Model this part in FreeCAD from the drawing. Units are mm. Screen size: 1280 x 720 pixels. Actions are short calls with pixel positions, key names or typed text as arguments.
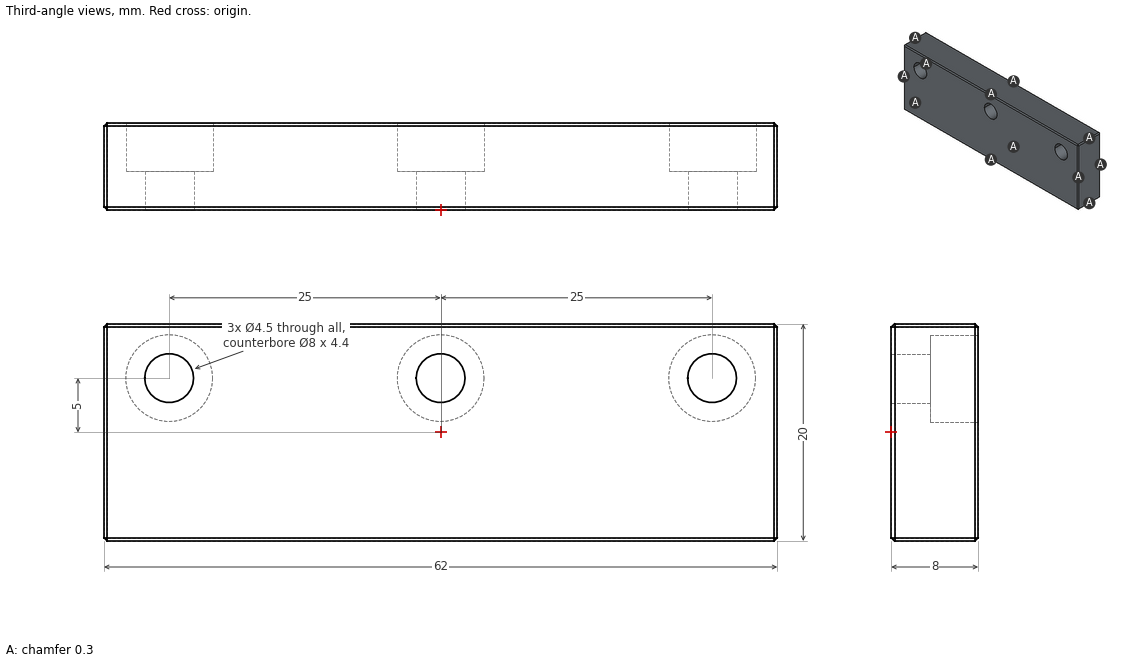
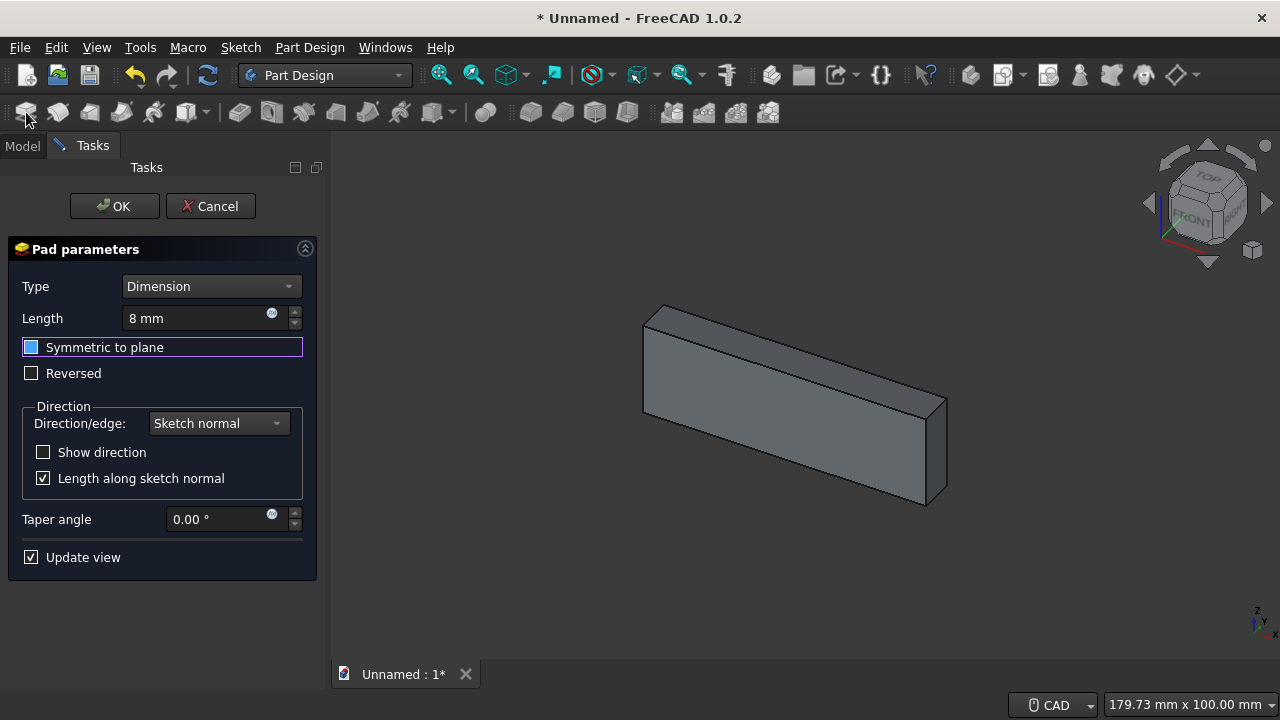
click(30, 373)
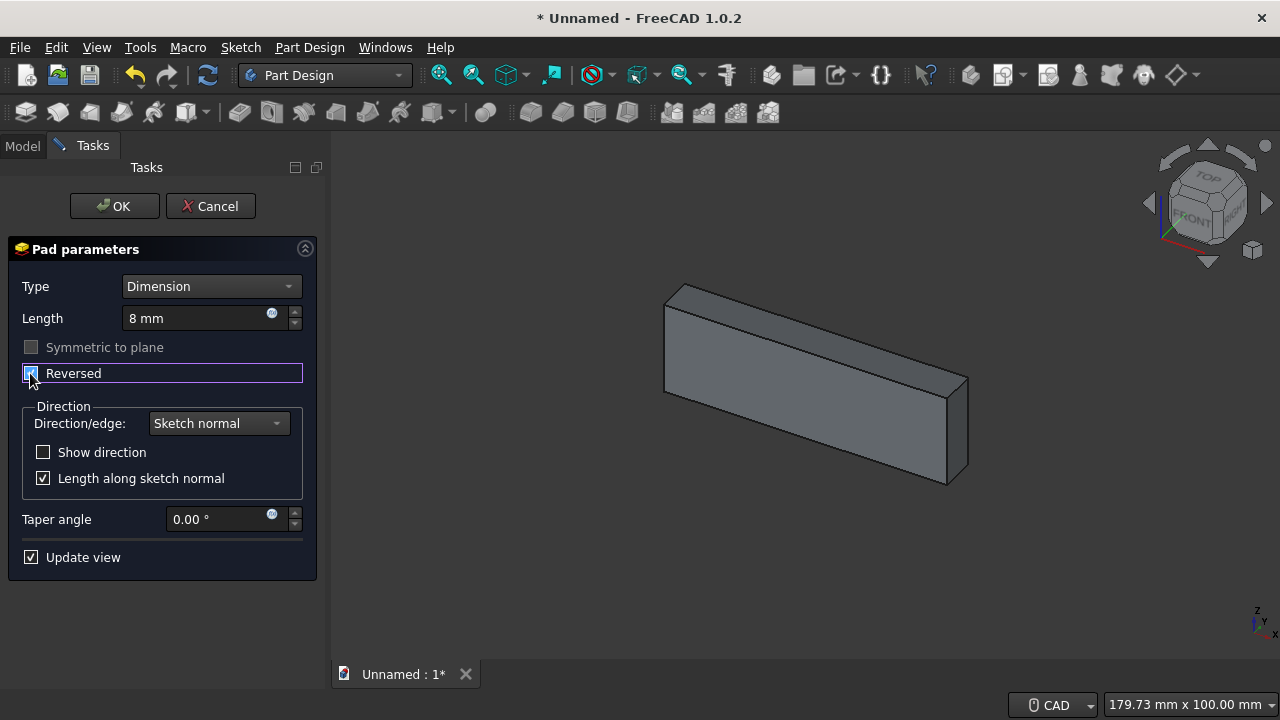
click(115, 206)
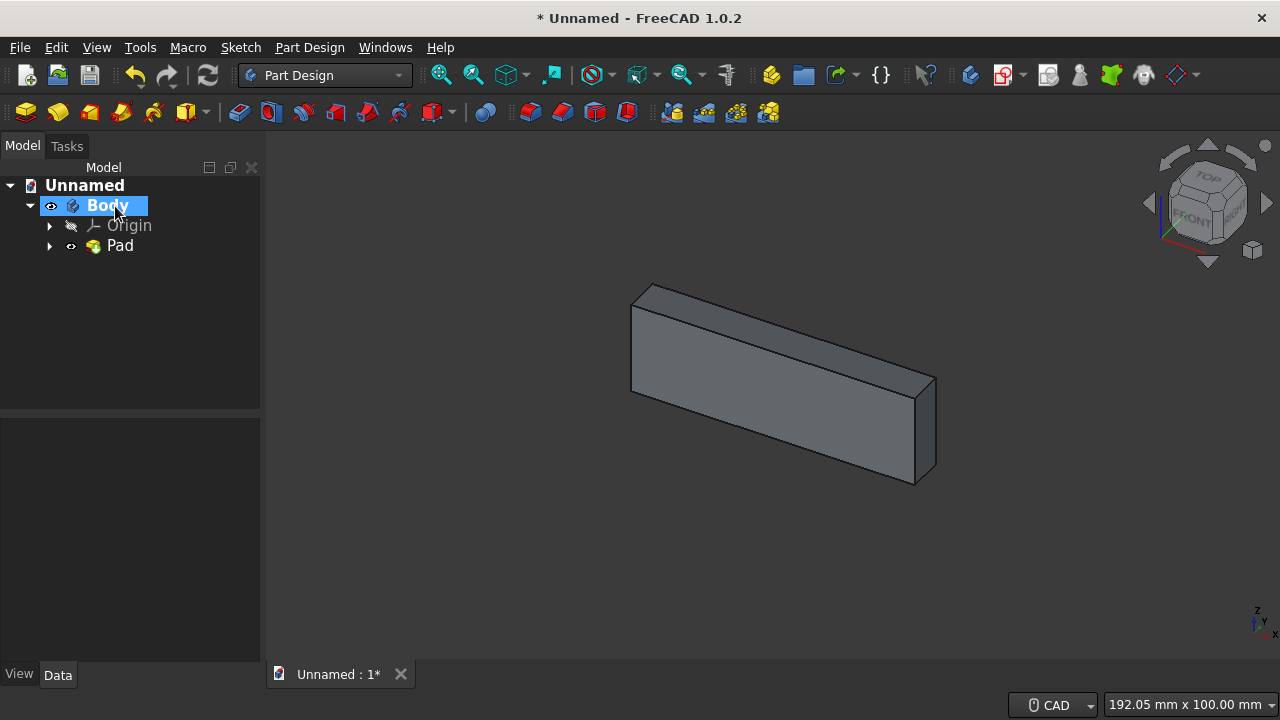
key(v)
key(f)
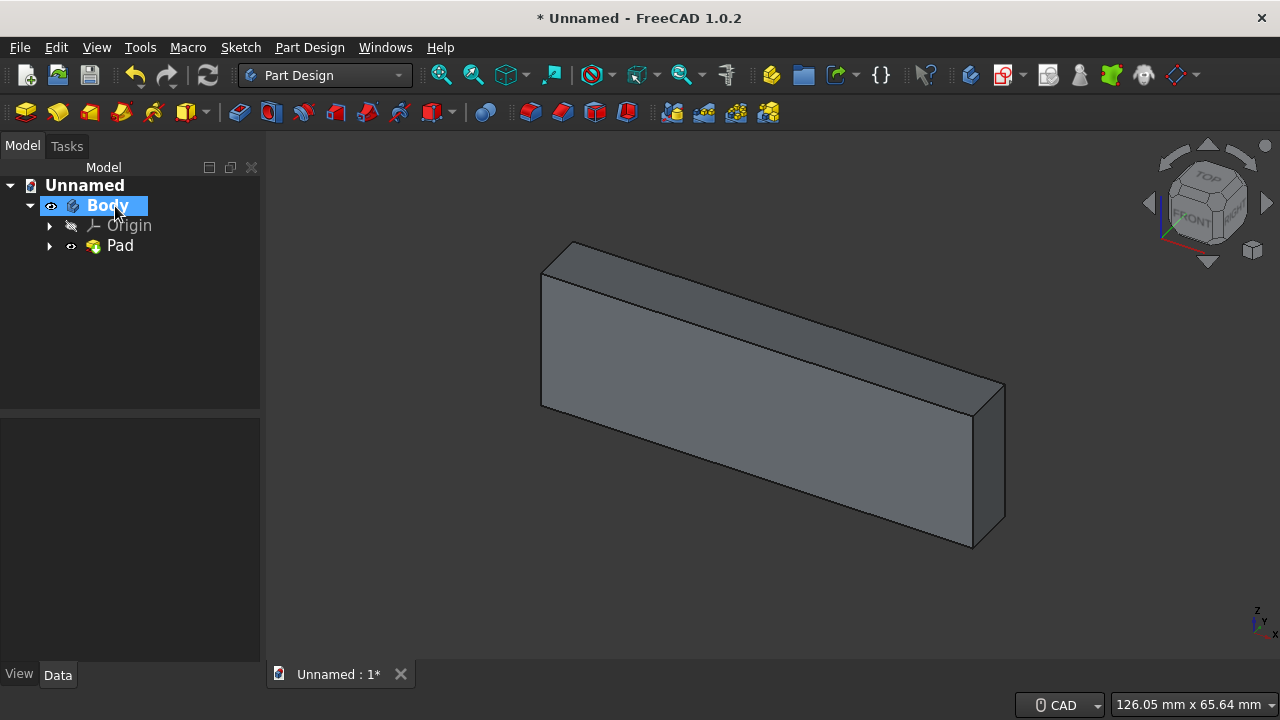
key(4)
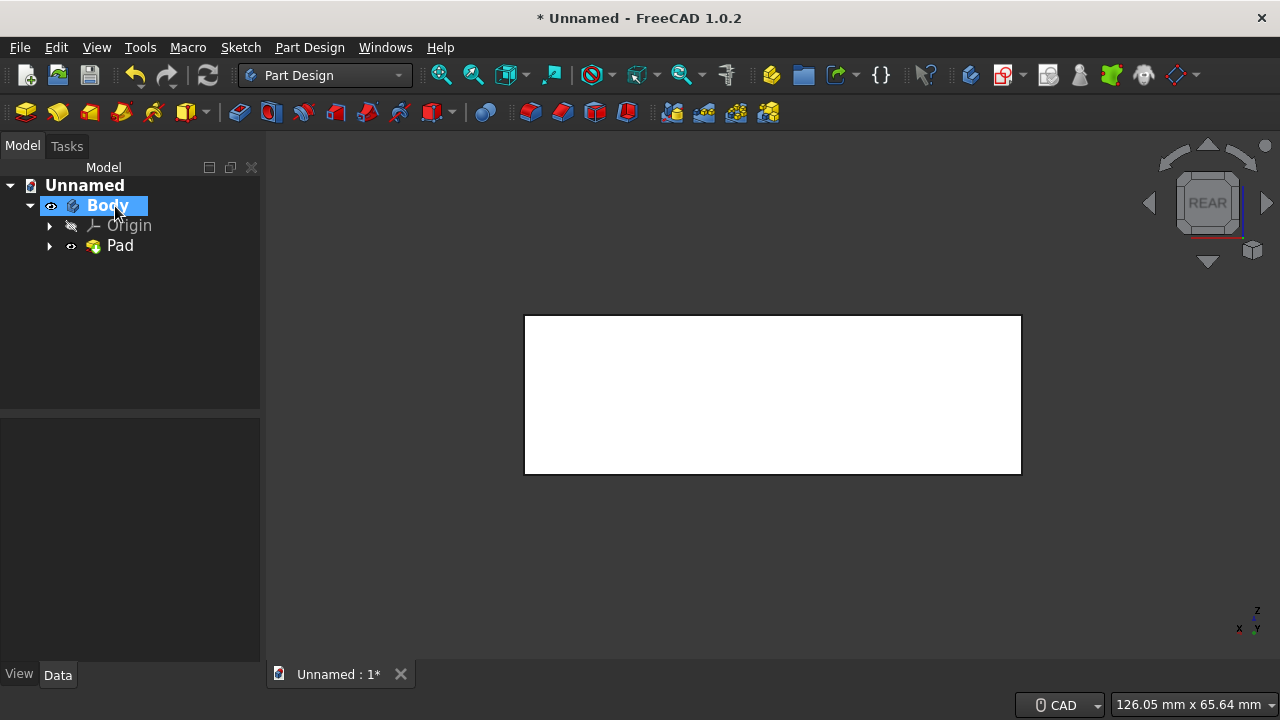
click(630, 394)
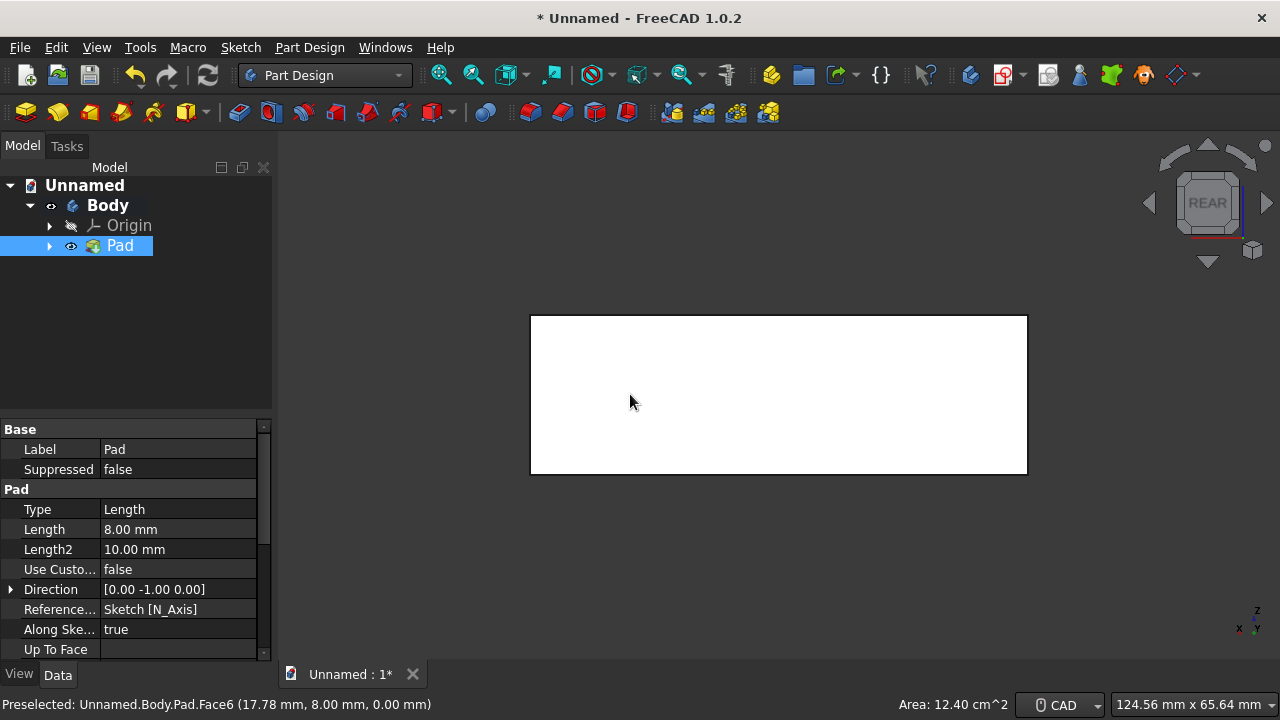
click(1004, 76)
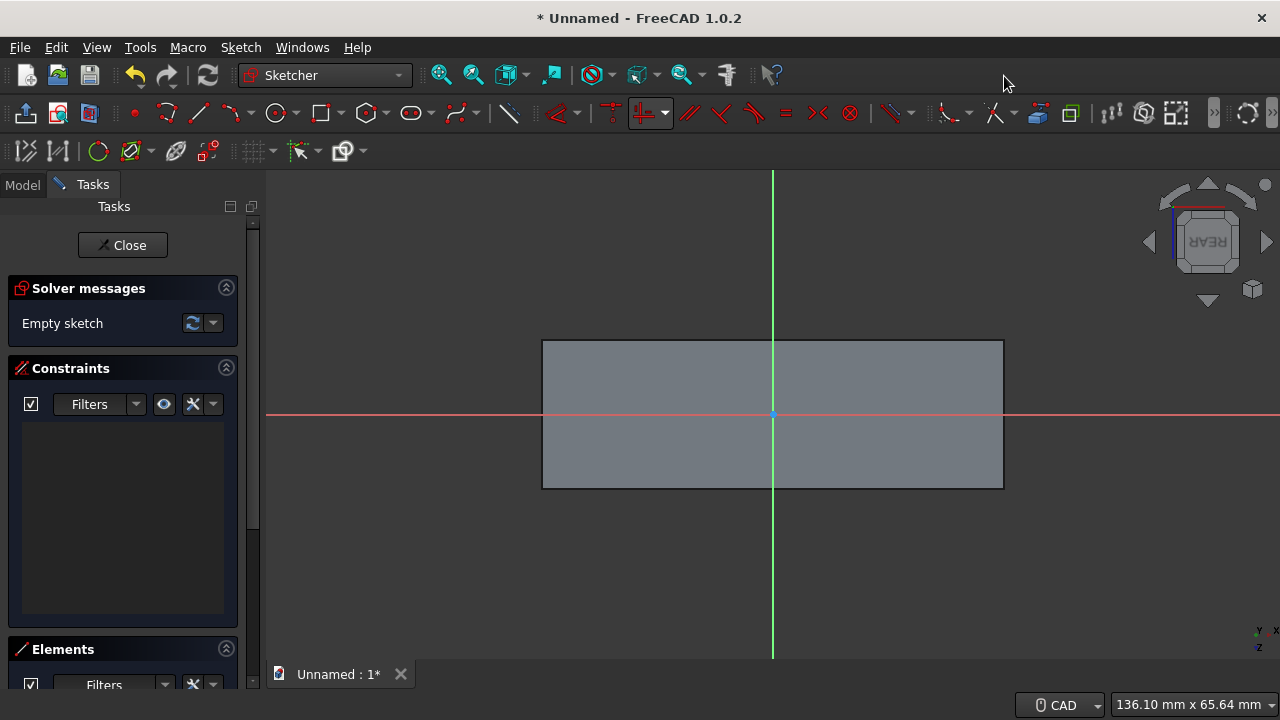
scroll(912, 496, up, 2)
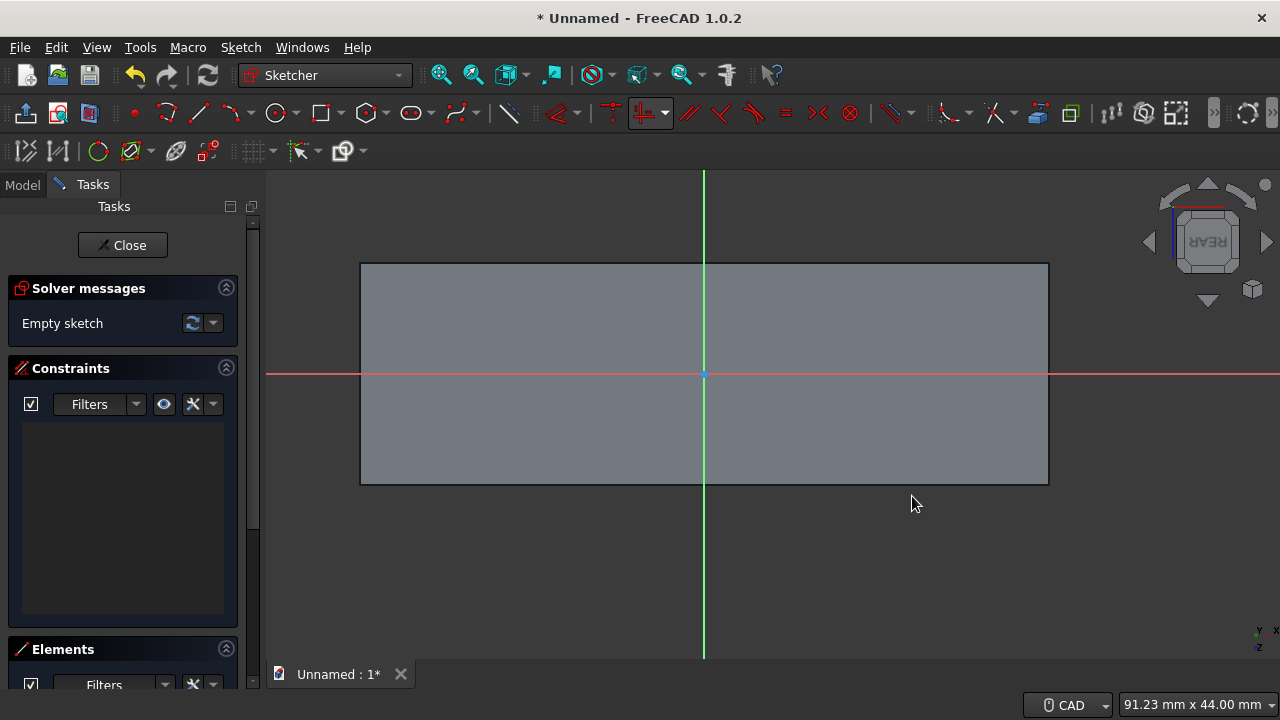
key(g)
key(c)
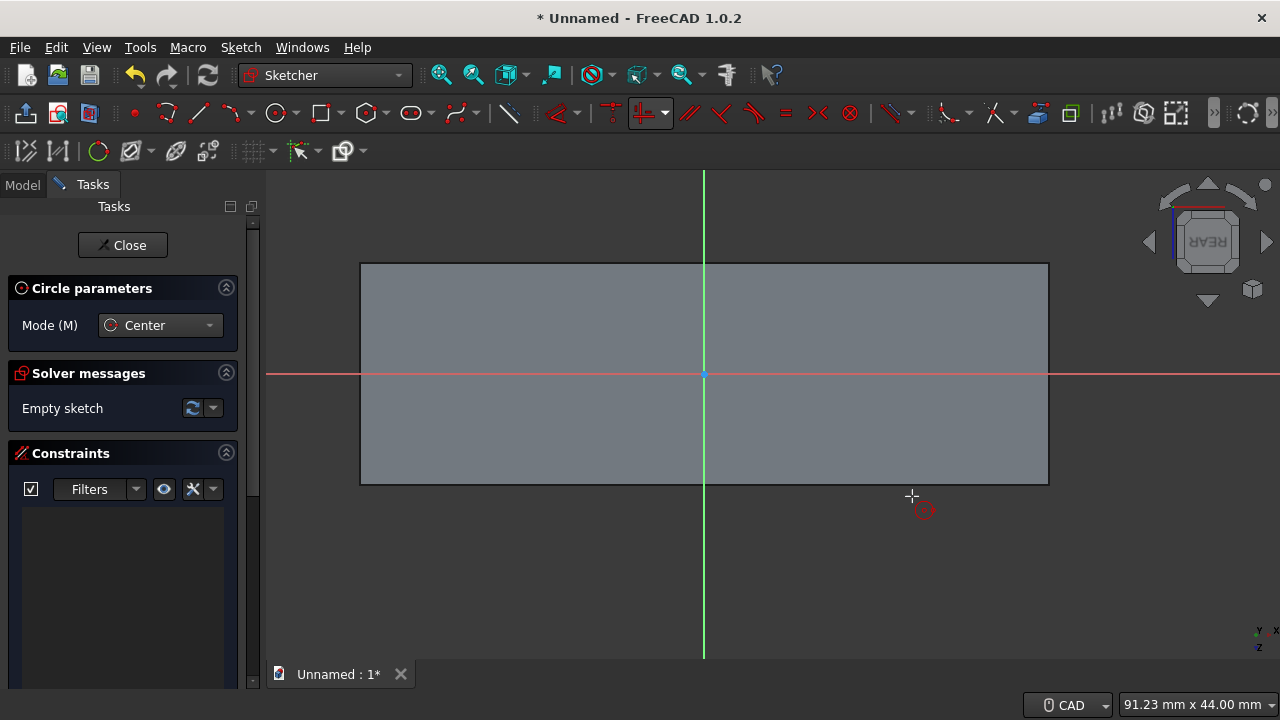
click(426, 430)
move(444, 412)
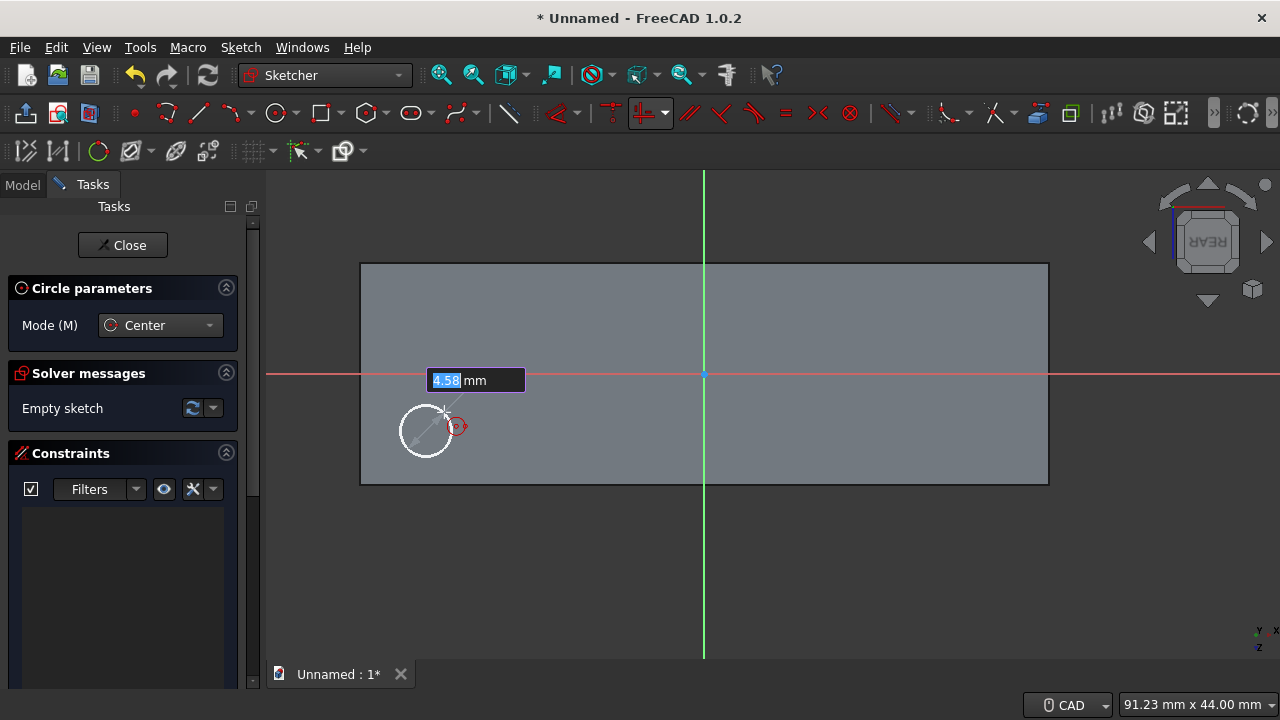
text(4.5)
key(Return)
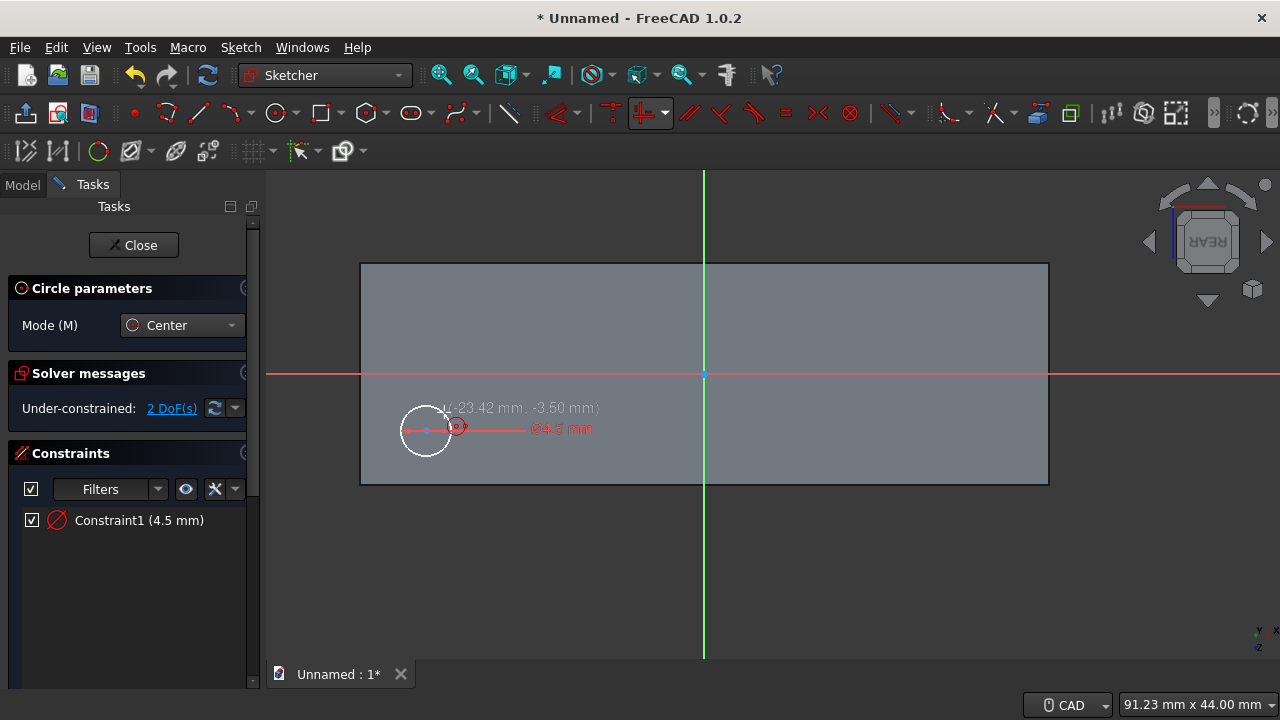
click(704, 430)
move(722, 412)